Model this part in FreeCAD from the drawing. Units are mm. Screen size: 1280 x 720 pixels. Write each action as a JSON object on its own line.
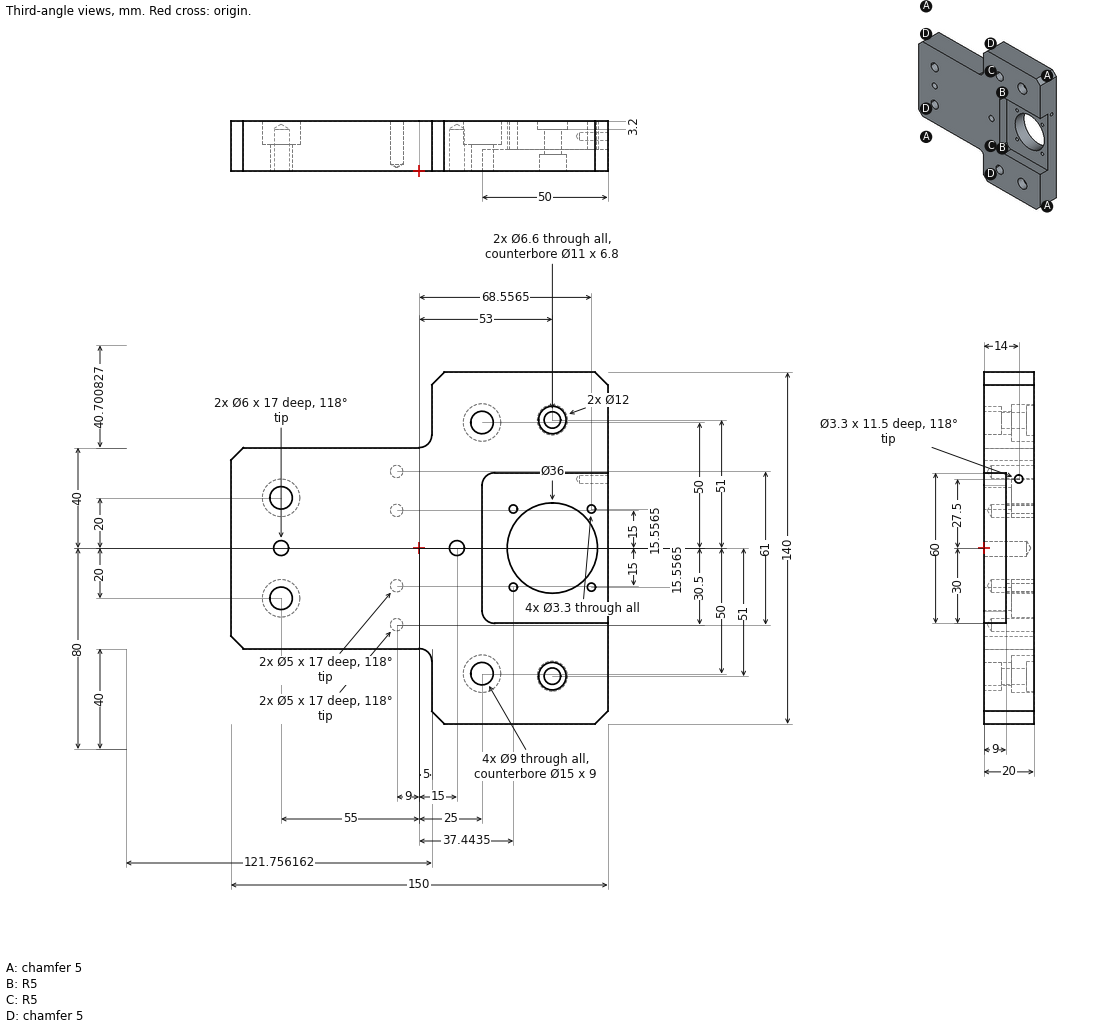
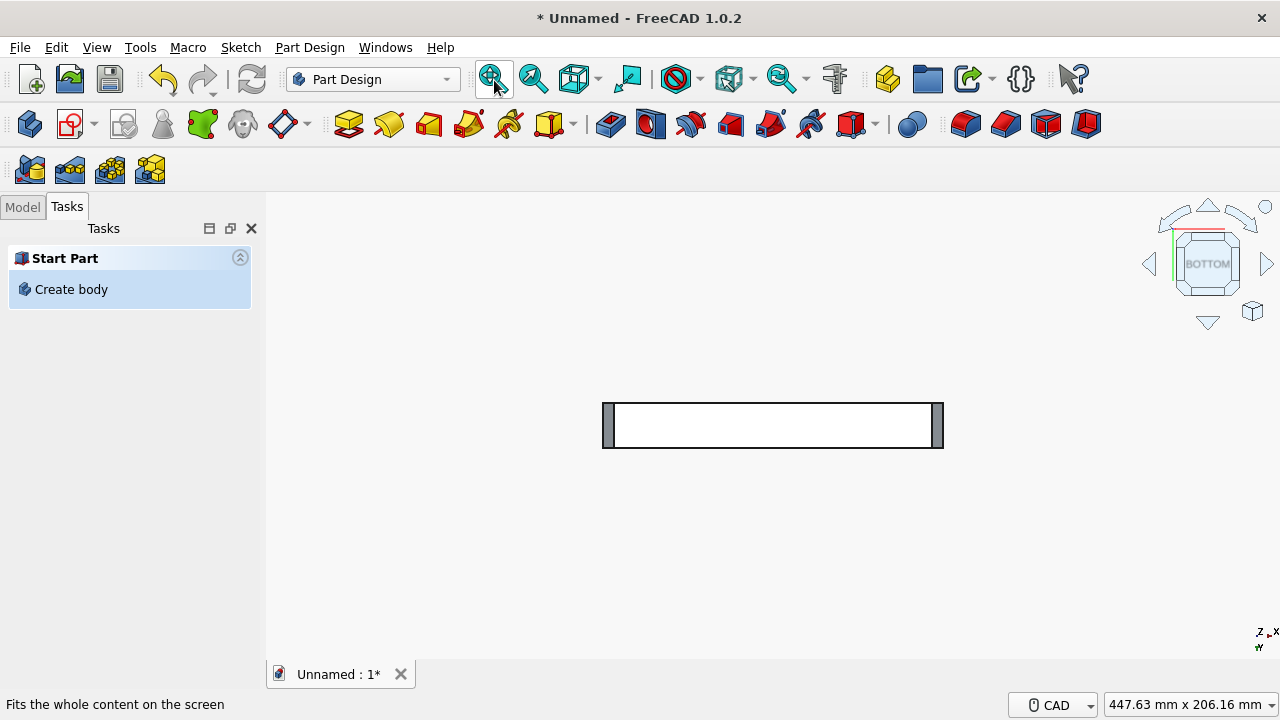
{"action": "left_click", "coordinate": [494, 80]}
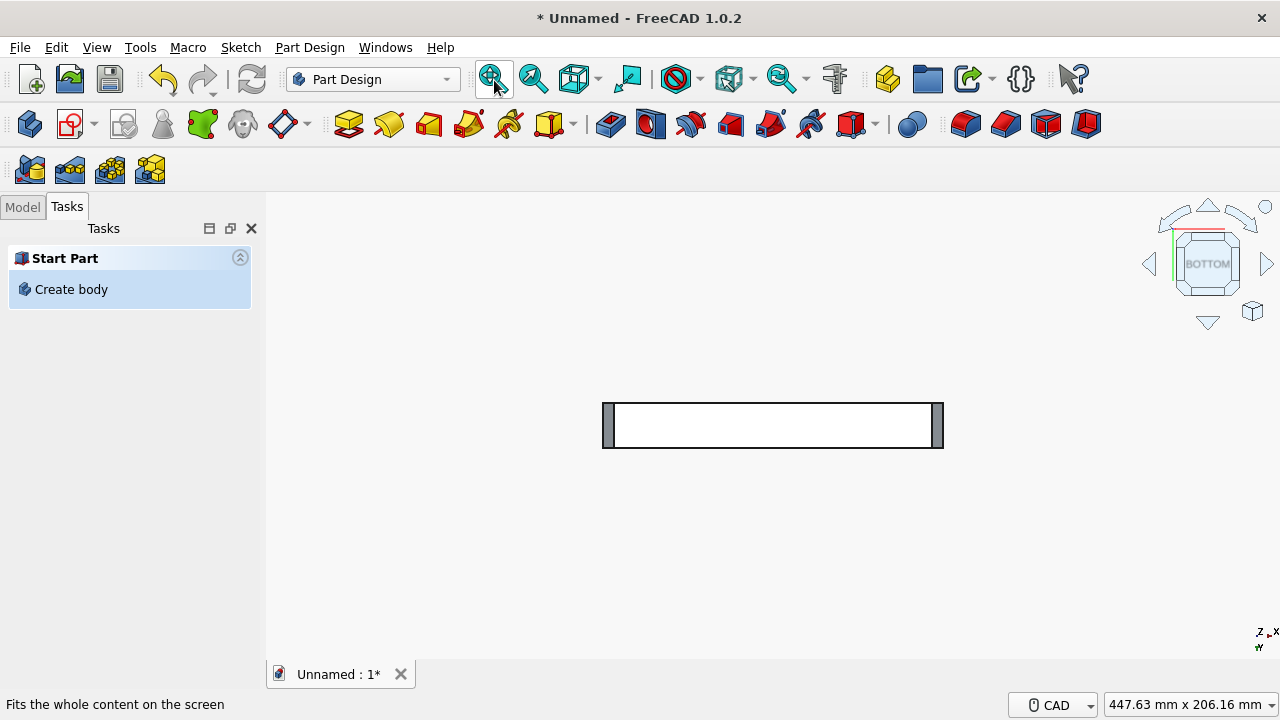
{"action": "scroll", "coordinate": [830, 412], "scroll_direction": "up", "scroll_amount": 4}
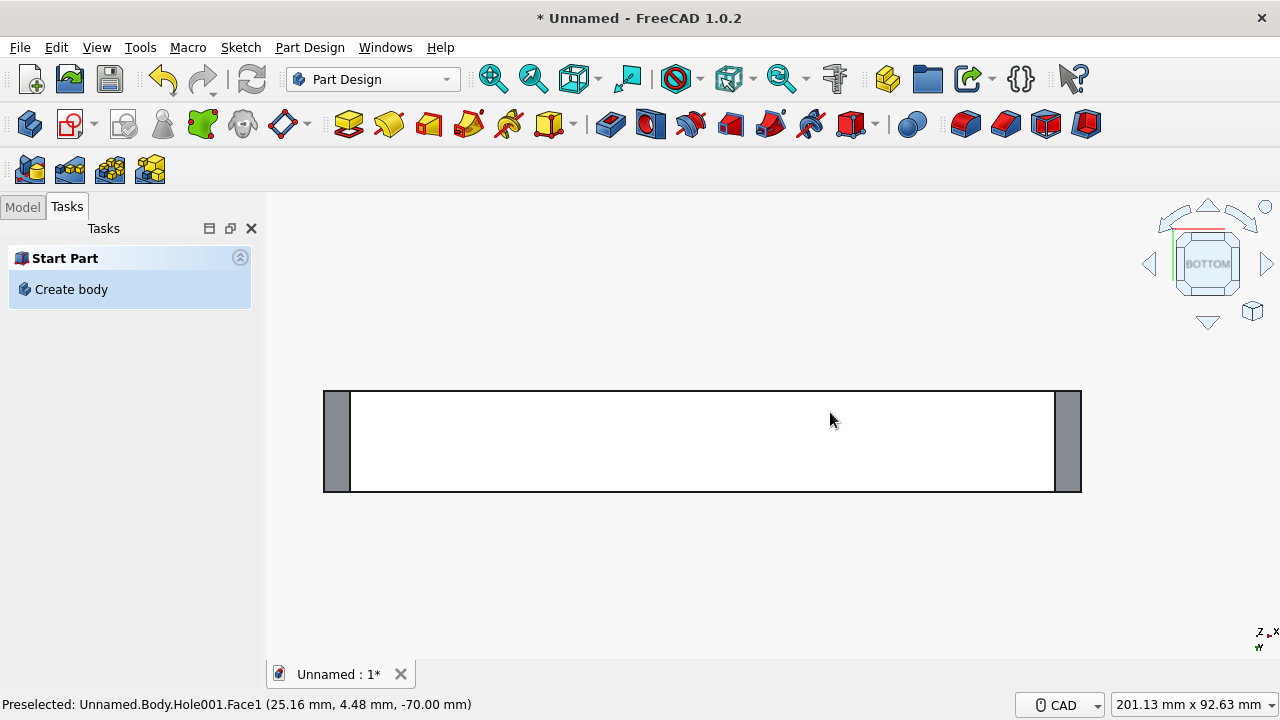
{"action": "left_click", "coordinate": [494, 80]}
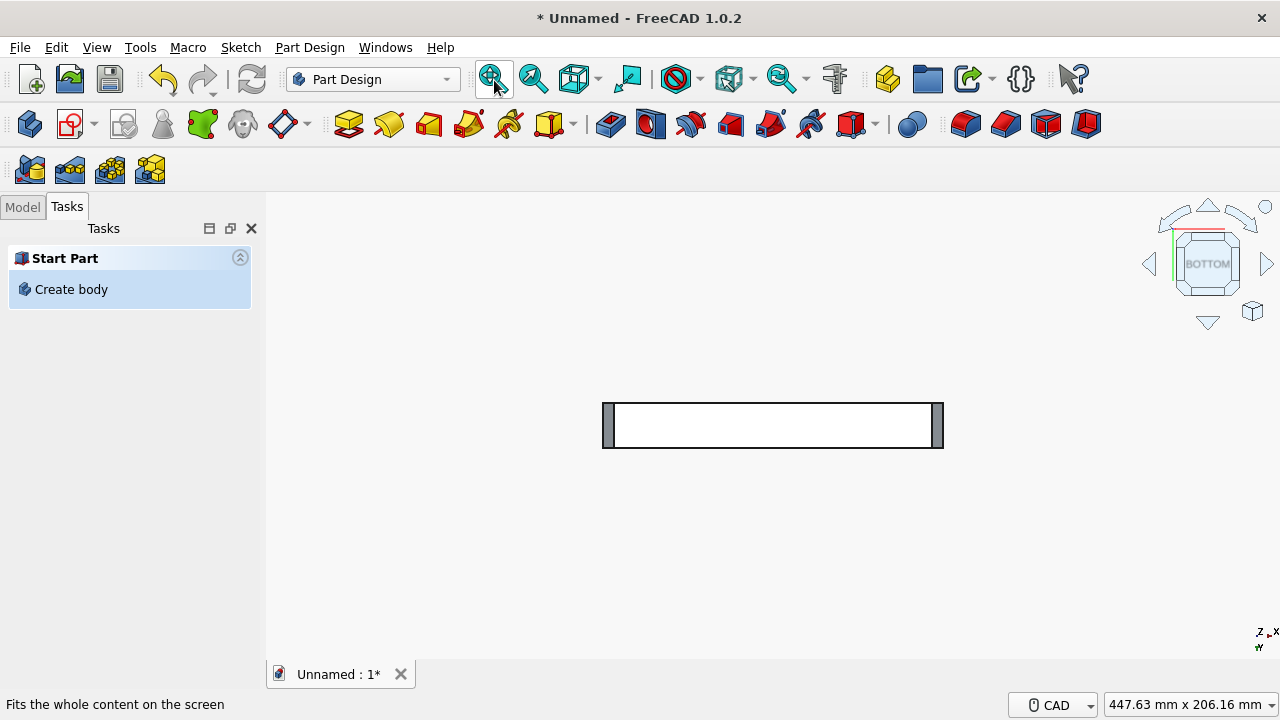
{"action": "key", "text": "4"}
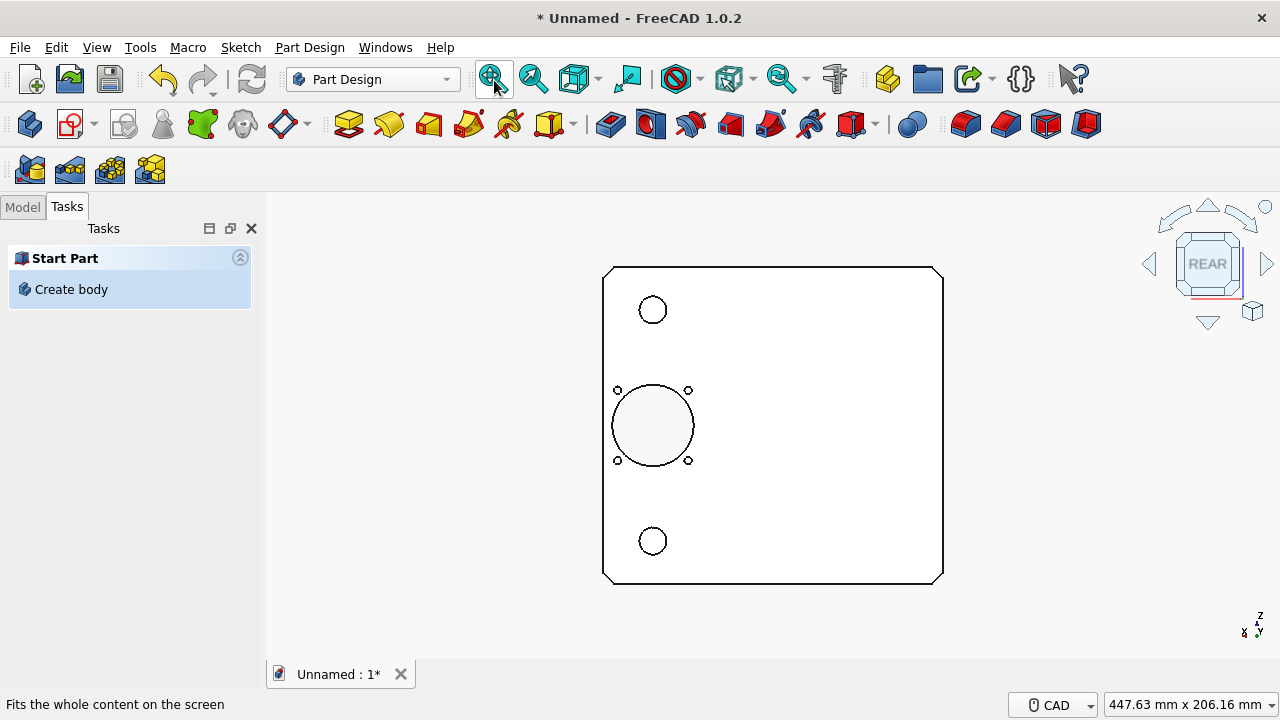
{"action": "scroll", "coordinate": [716, 357], "scroll_direction": "up", "scroll_amount": 4}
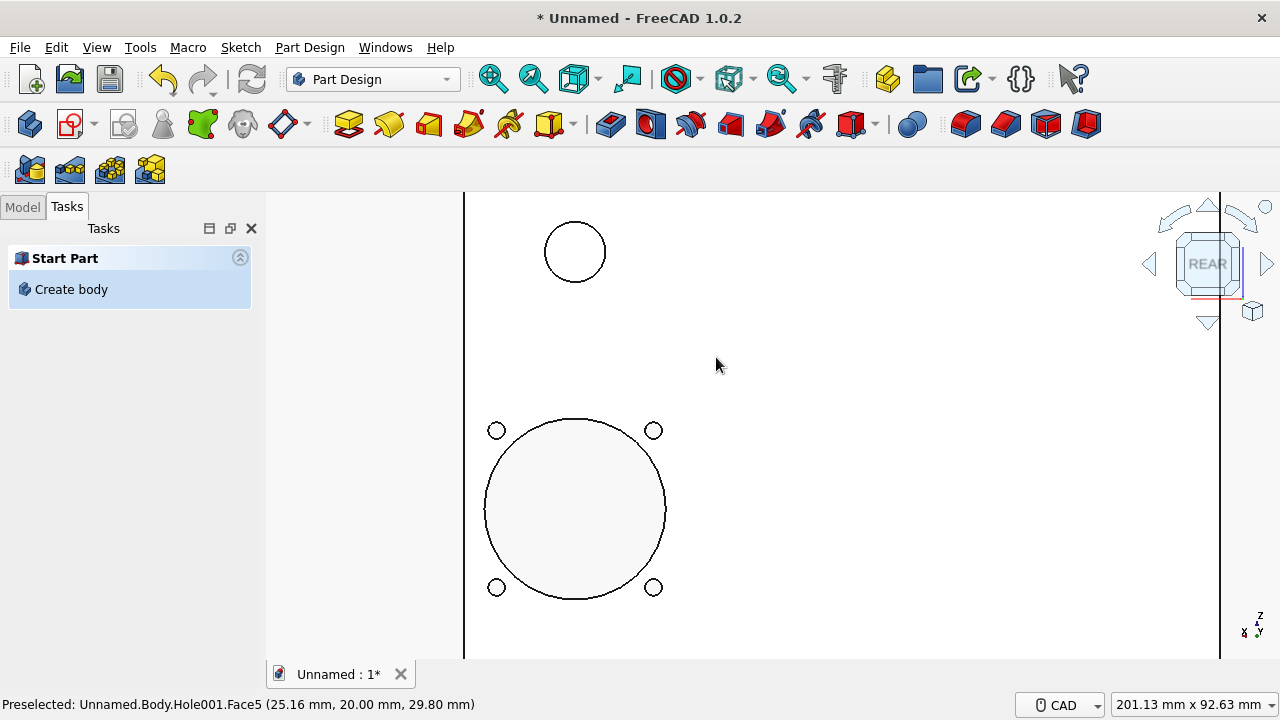
{"action": "left_click", "coordinate": [494, 80]}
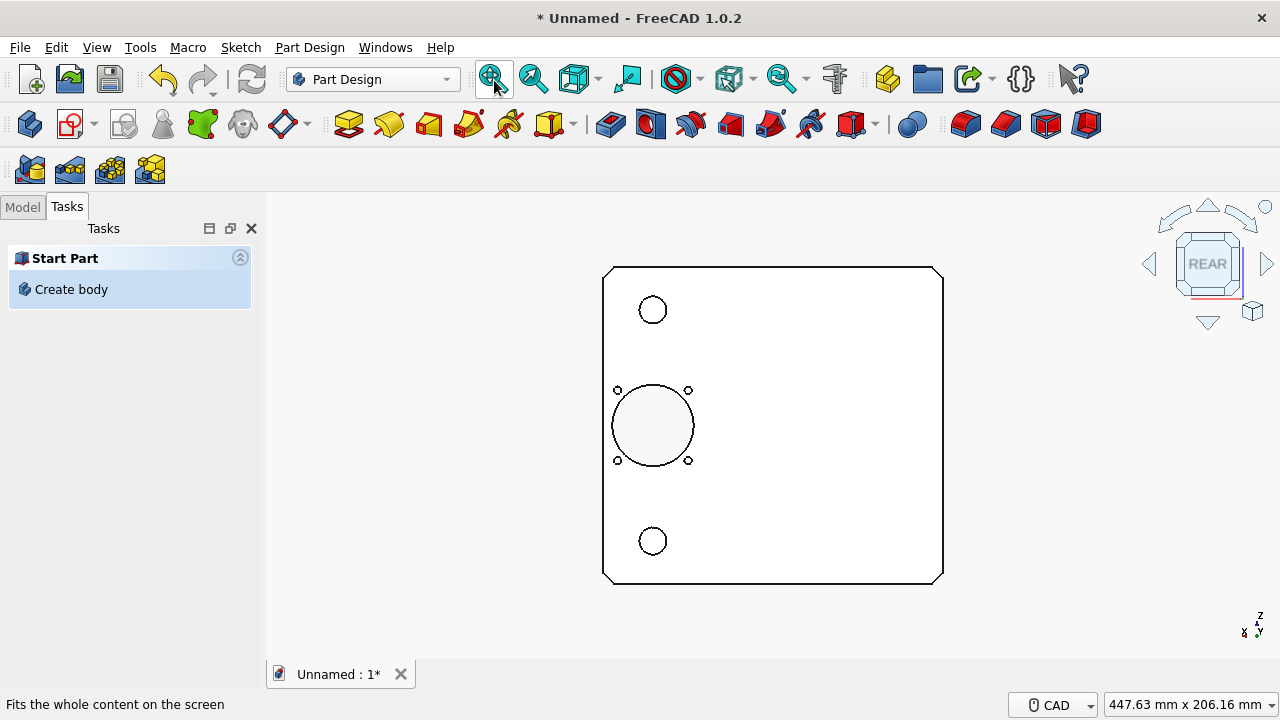
{"action": "key", "text": "6"}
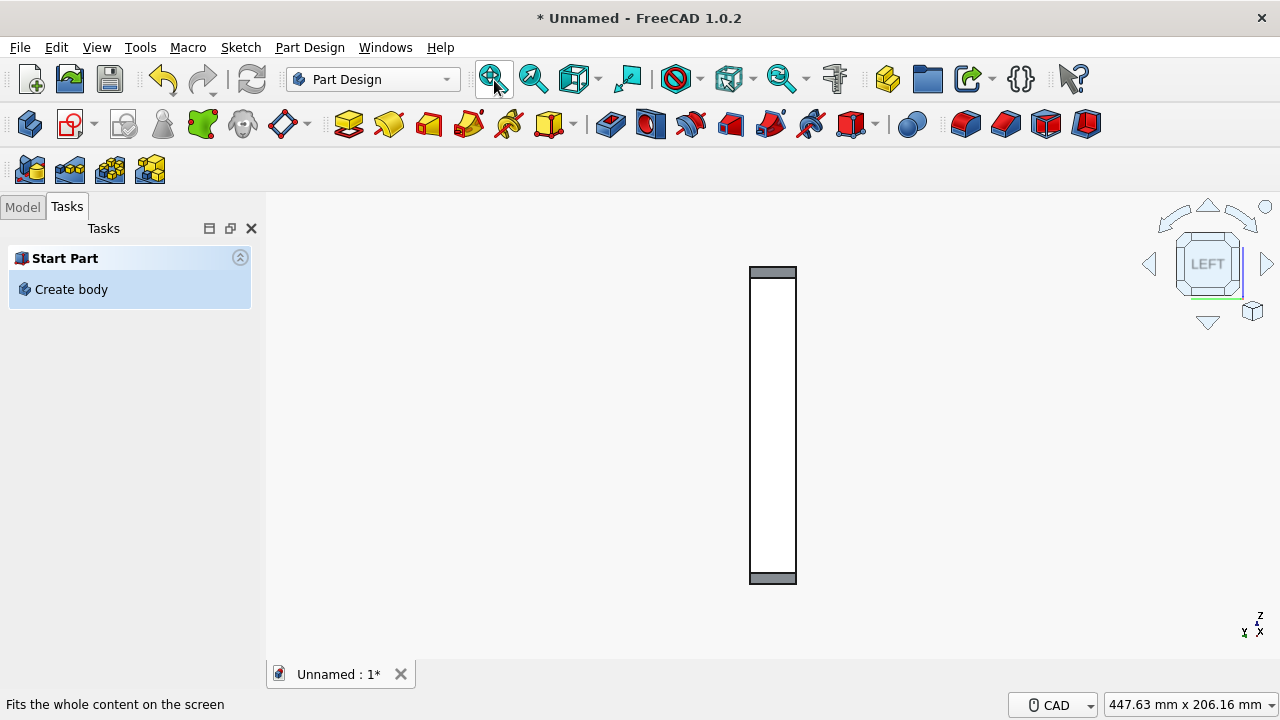
{"action": "scroll", "coordinate": [785, 357], "scroll_direction": "up", "scroll_amount": 4}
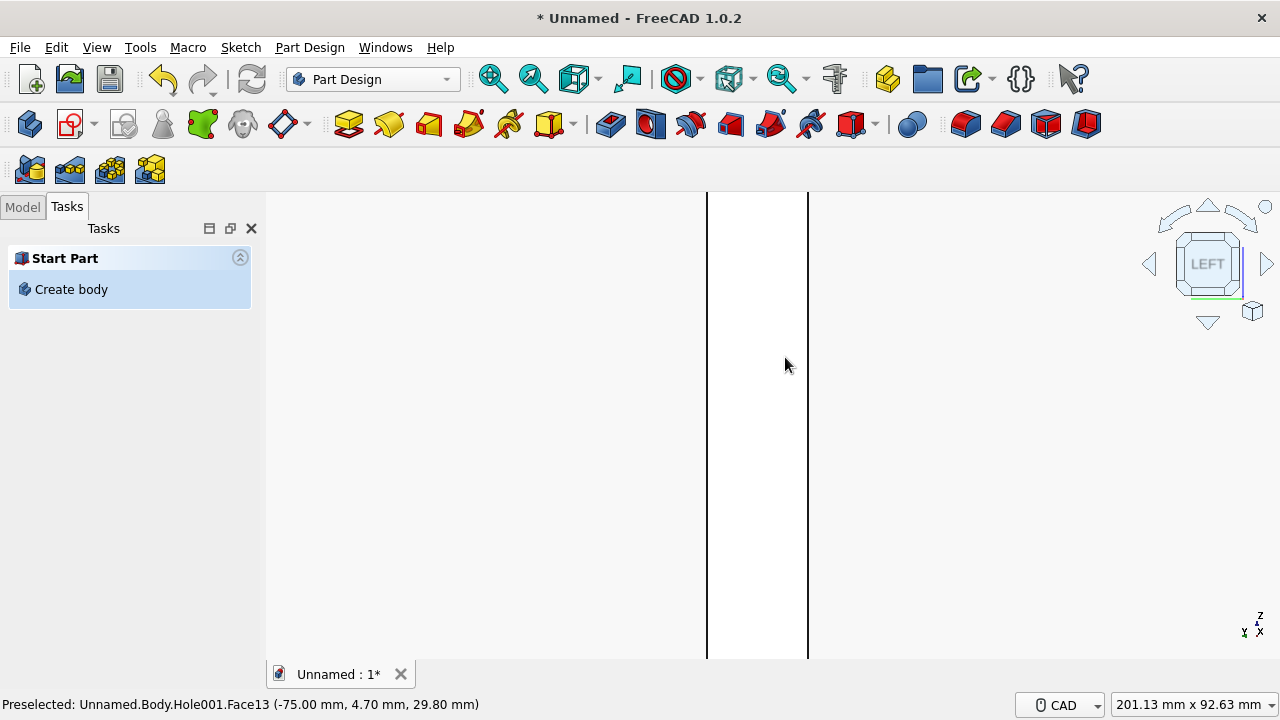
{"action": "left_click", "coordinate": [494, 80]}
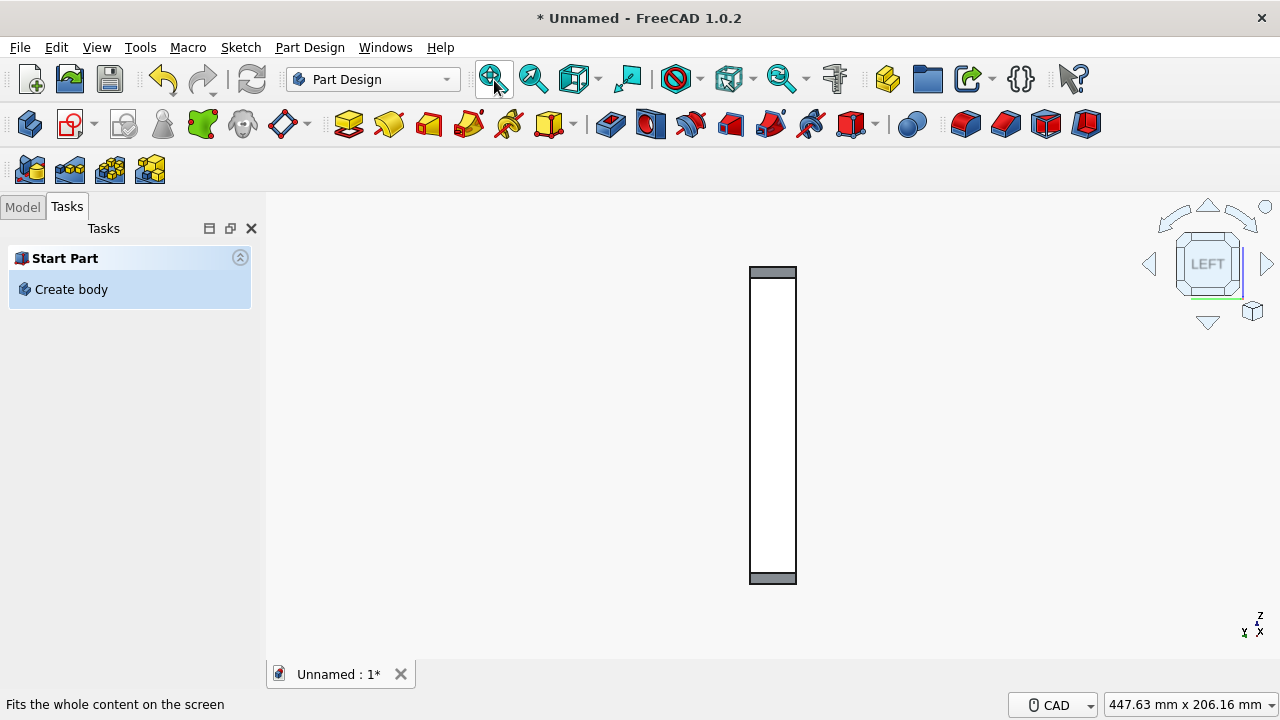
{"action": "key", "text": "v 3"}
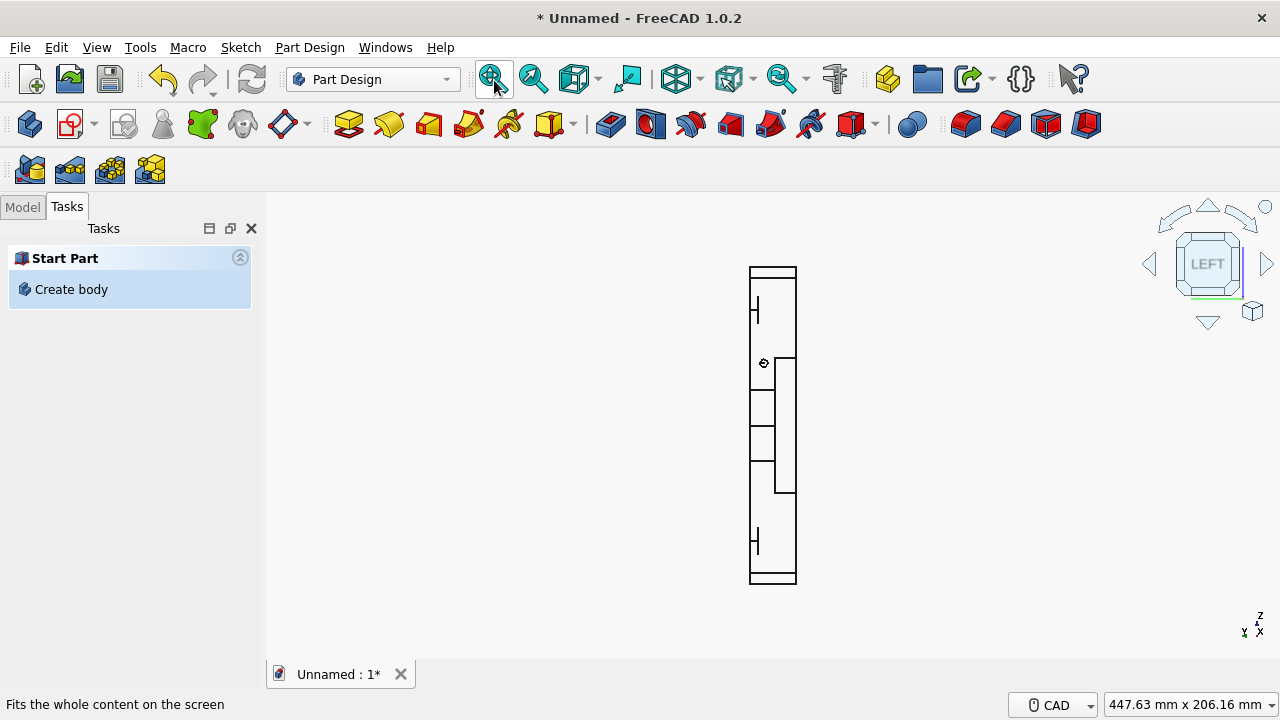
{"action": "key", "text": "0"}